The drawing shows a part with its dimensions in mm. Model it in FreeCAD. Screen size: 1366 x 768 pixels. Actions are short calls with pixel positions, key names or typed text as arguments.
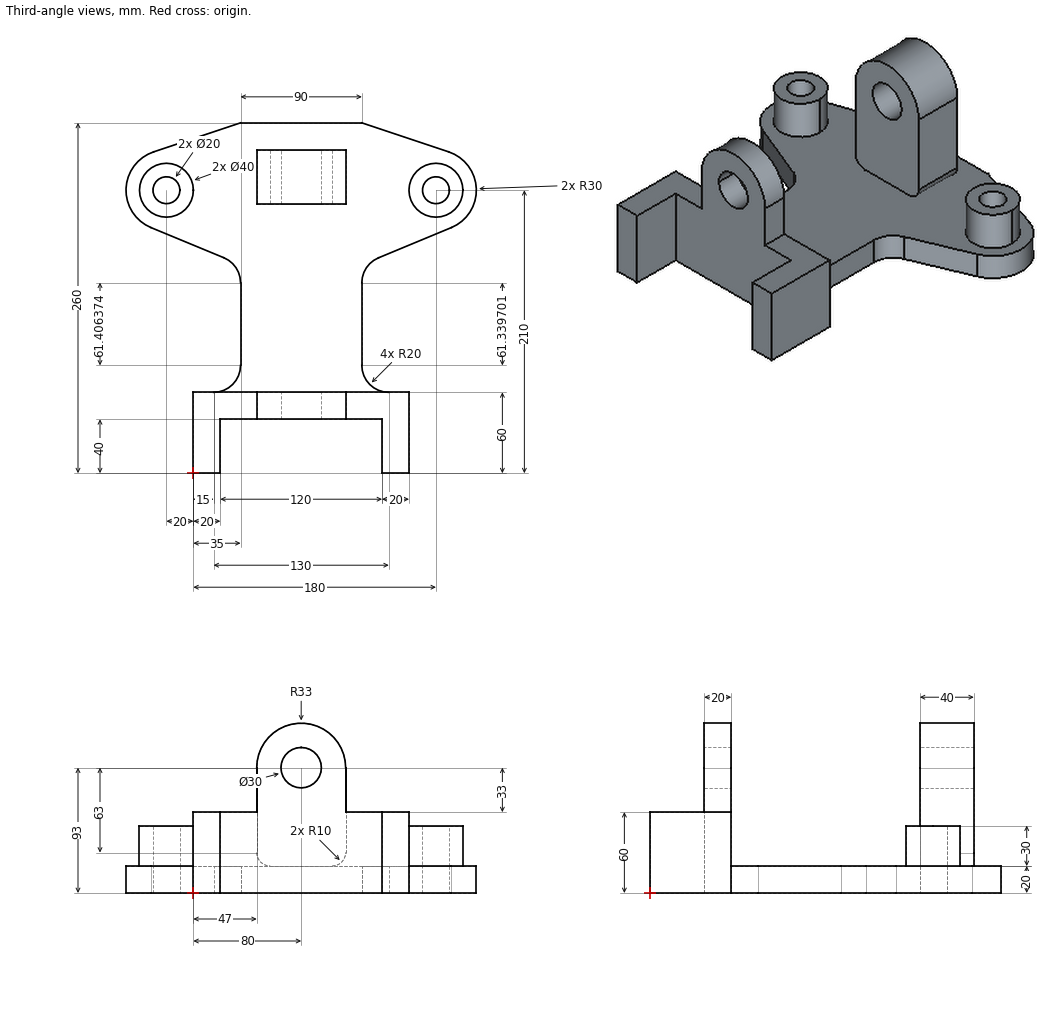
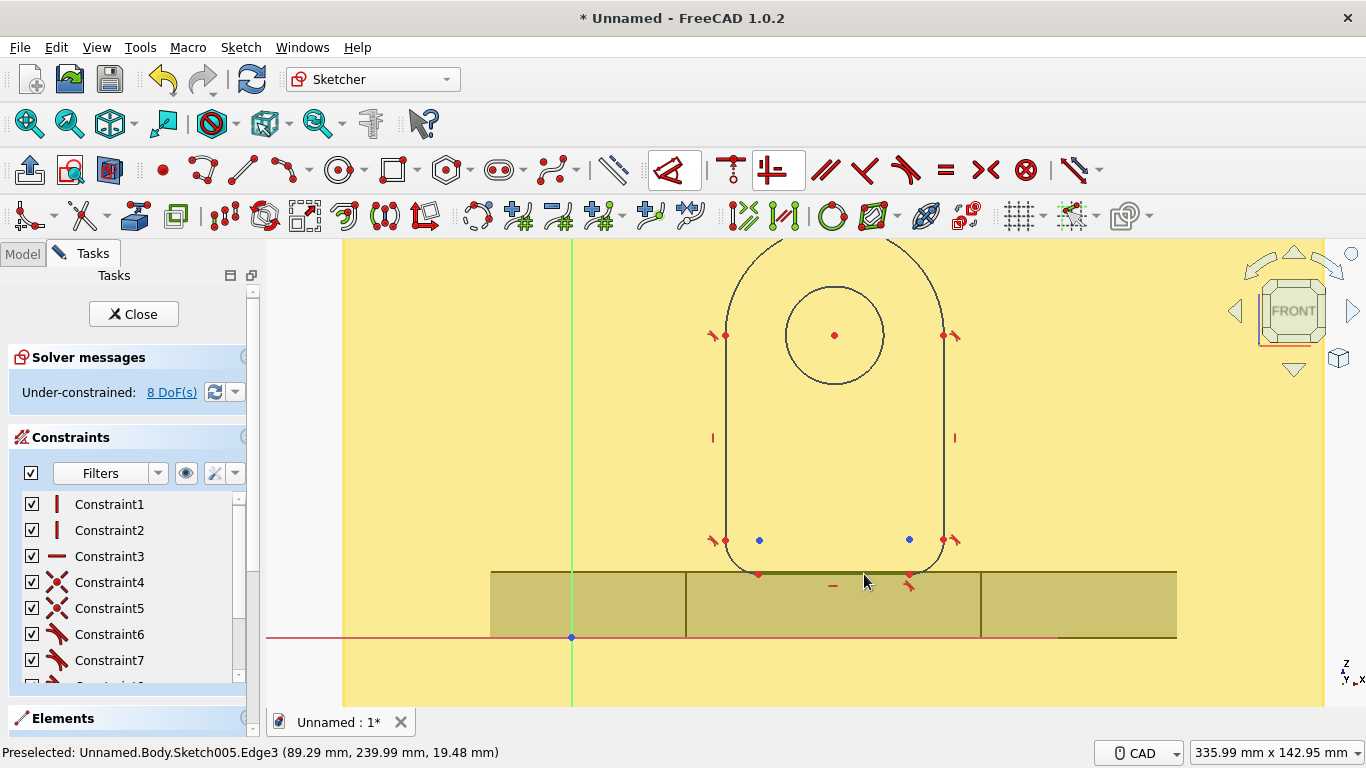
click(729, 555)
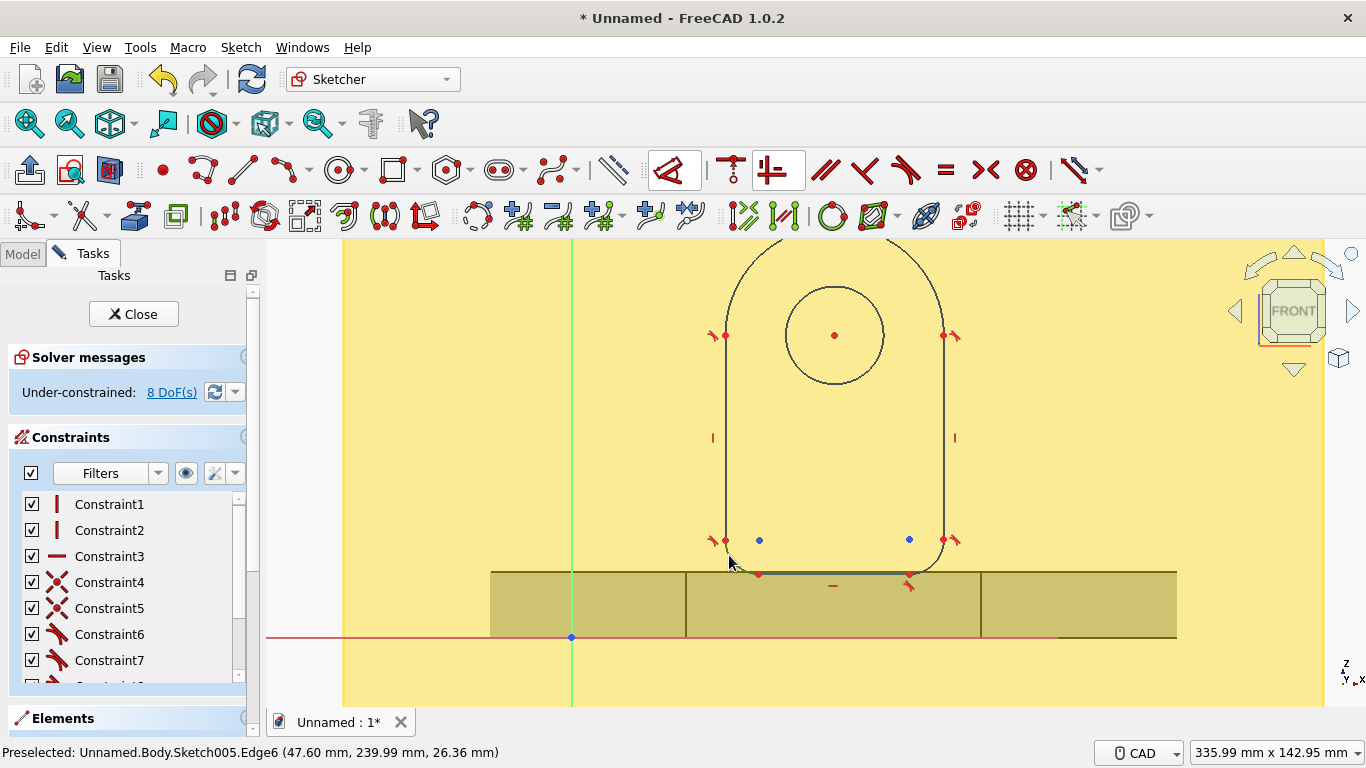
key(t)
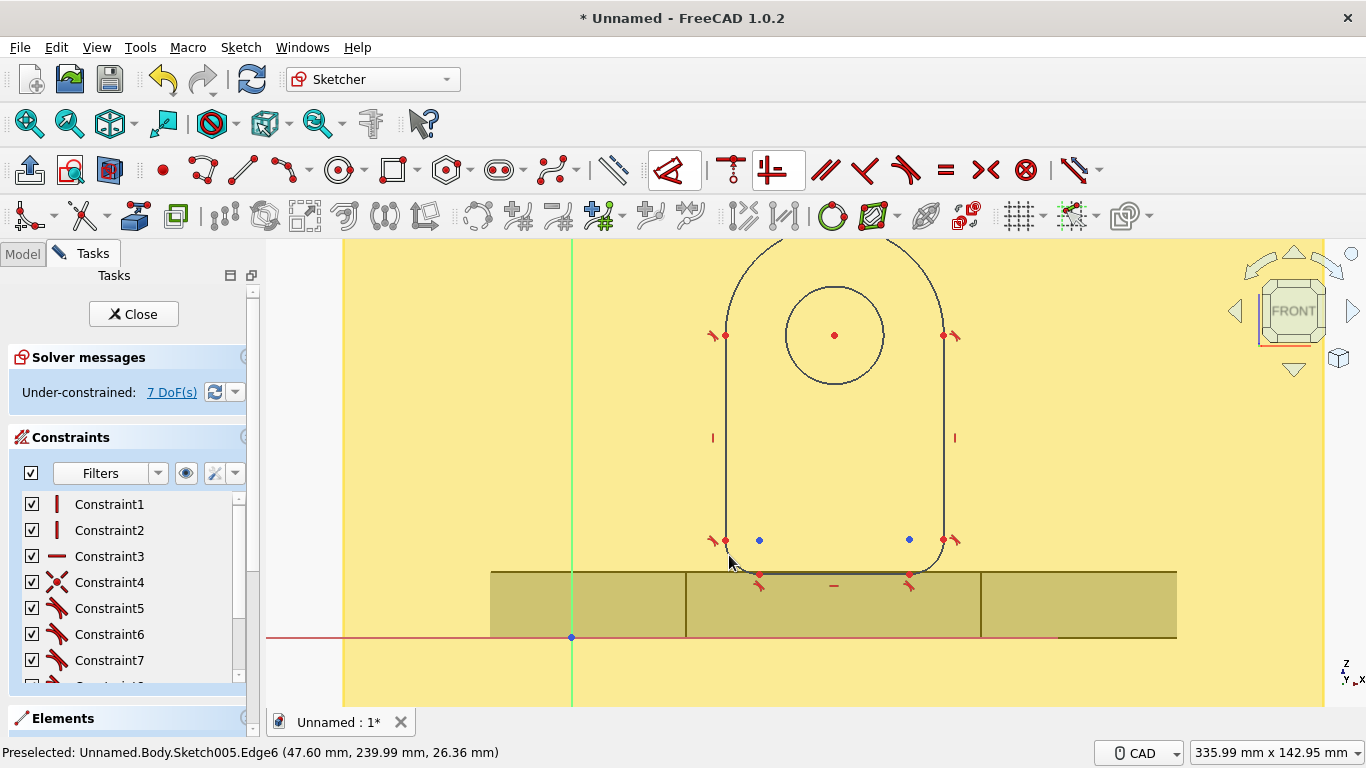
click(925, 570)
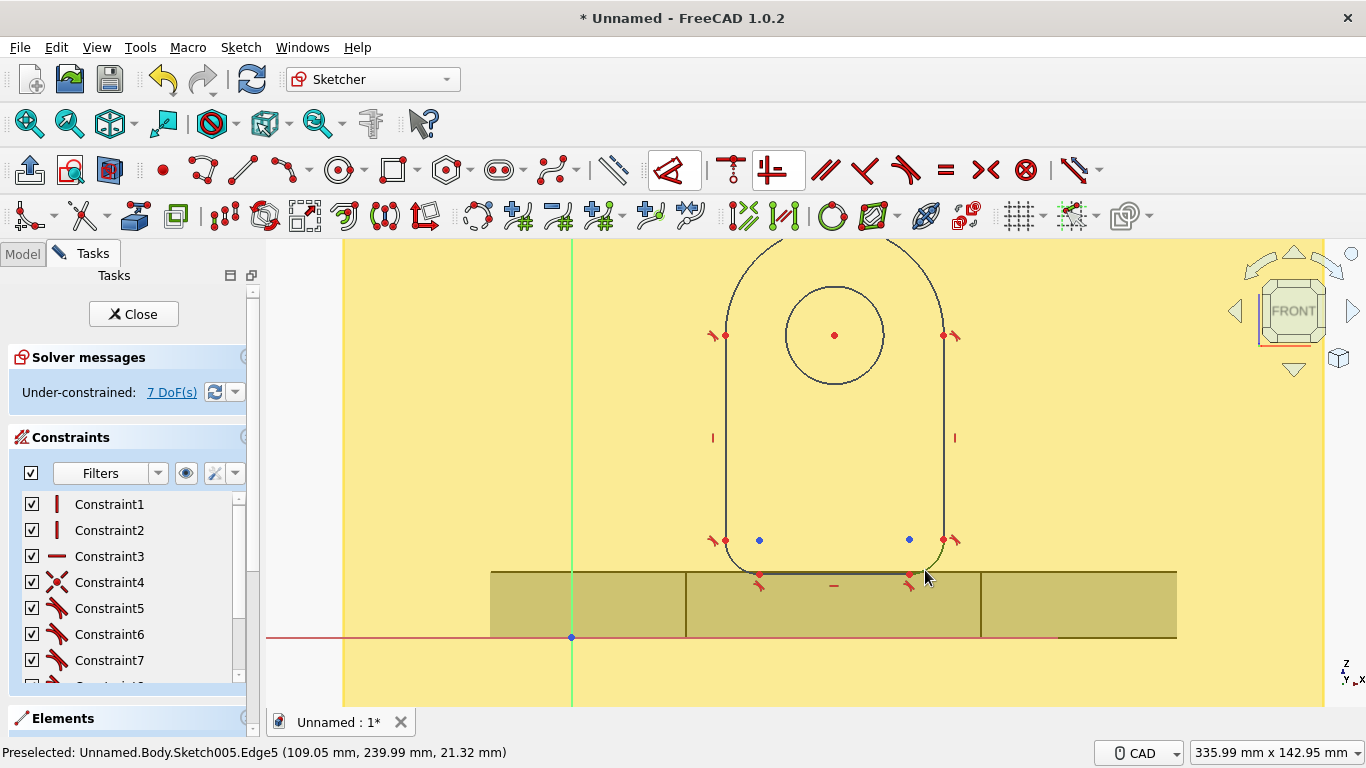
click(729, 556)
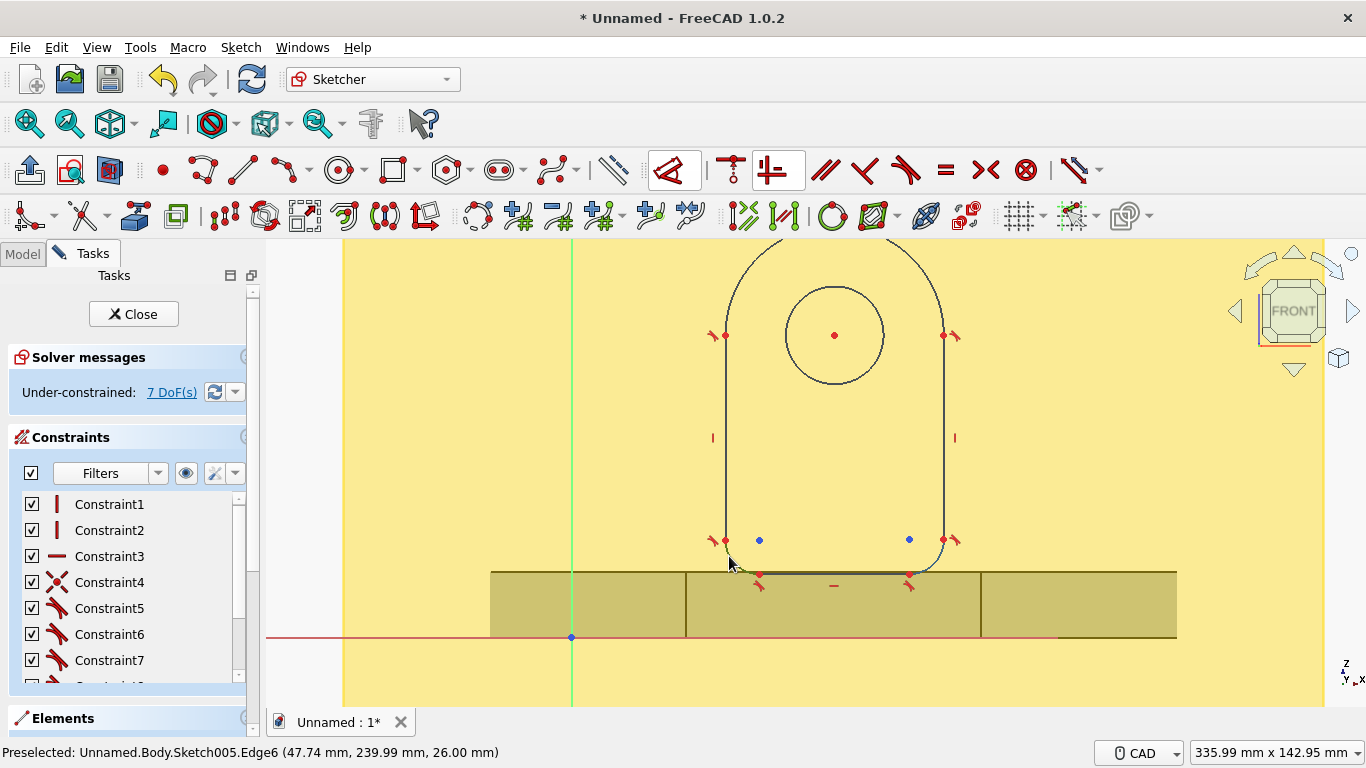
click(946, 170)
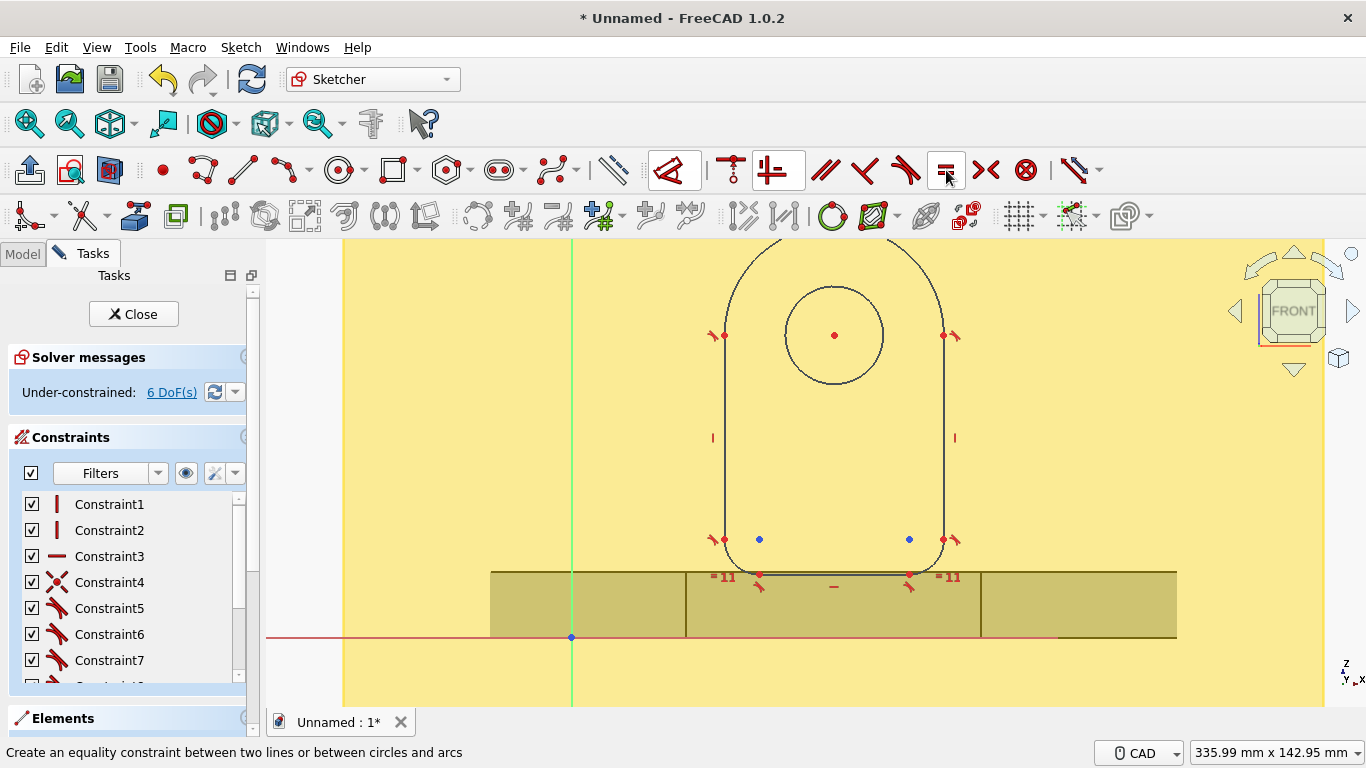
click(923, 271)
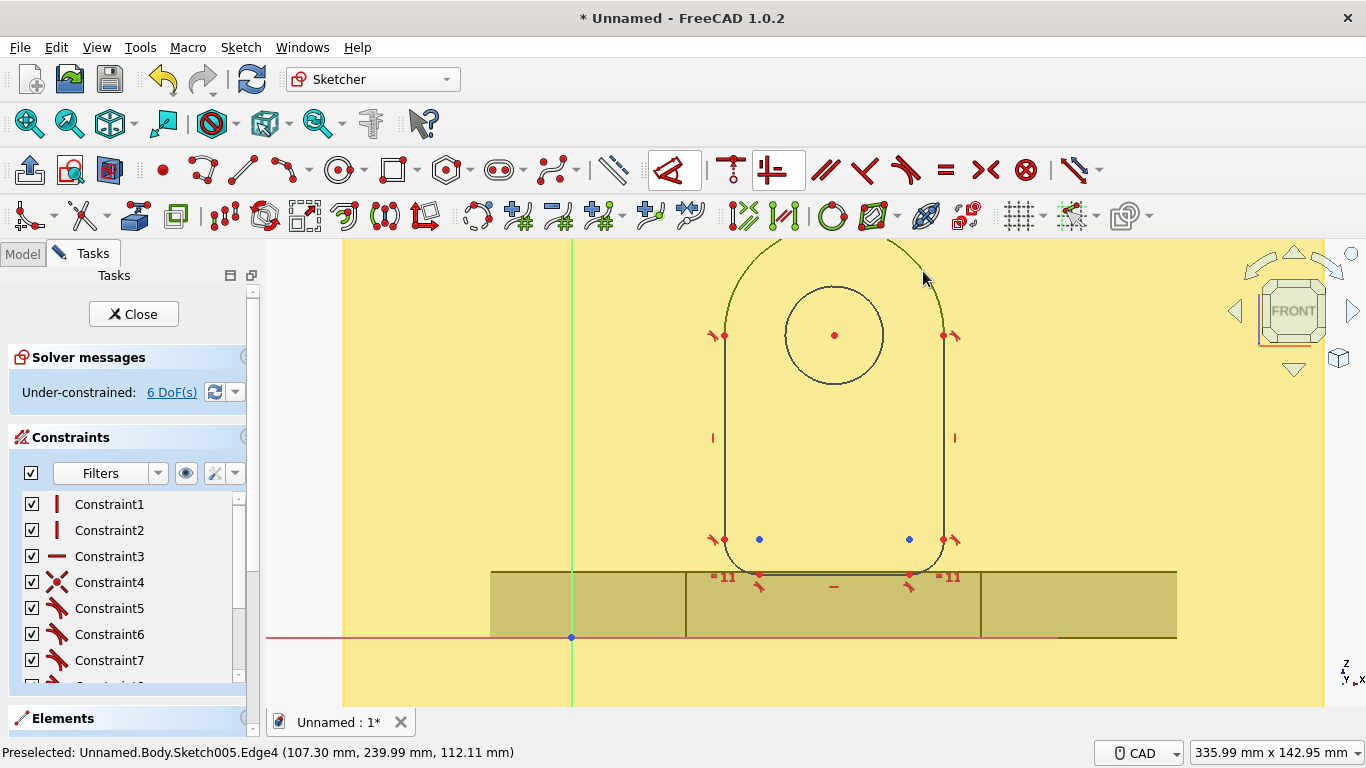
click(696, 170)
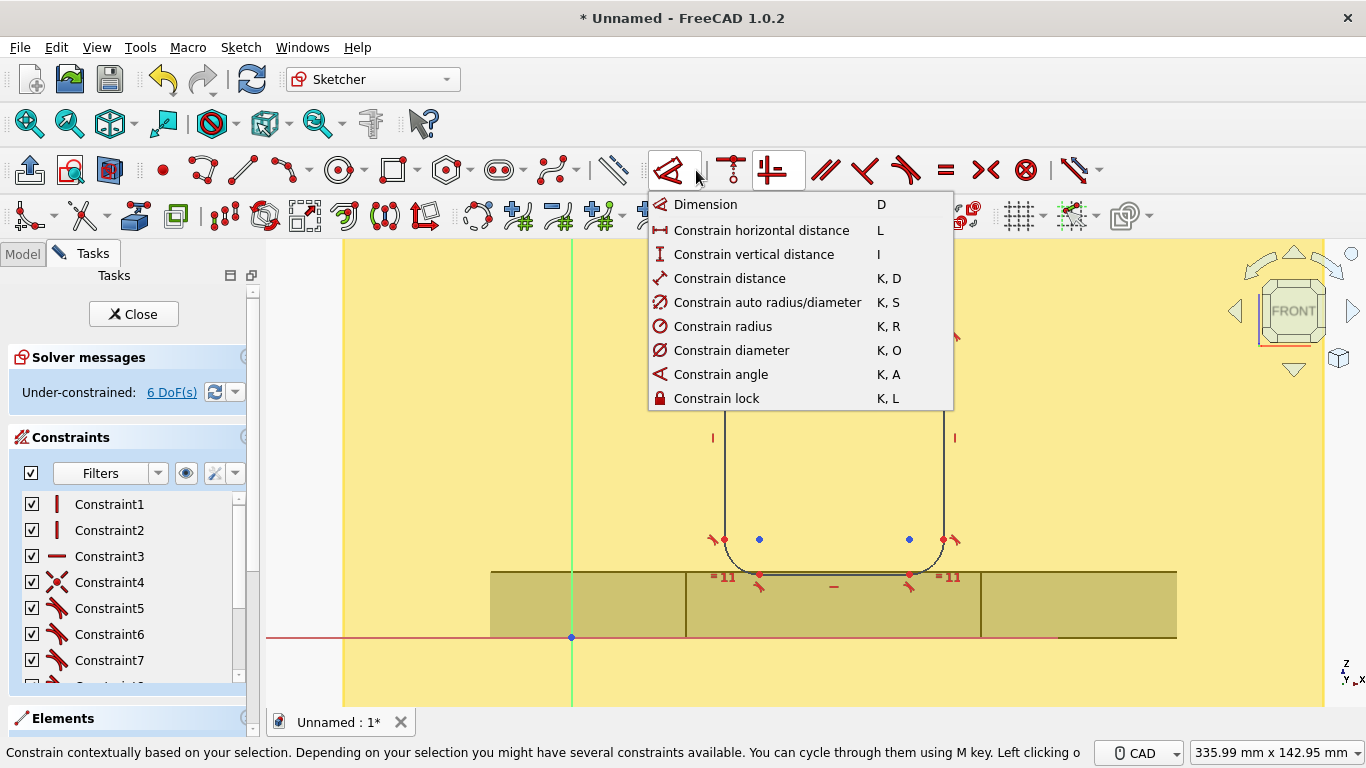
click(801, 326)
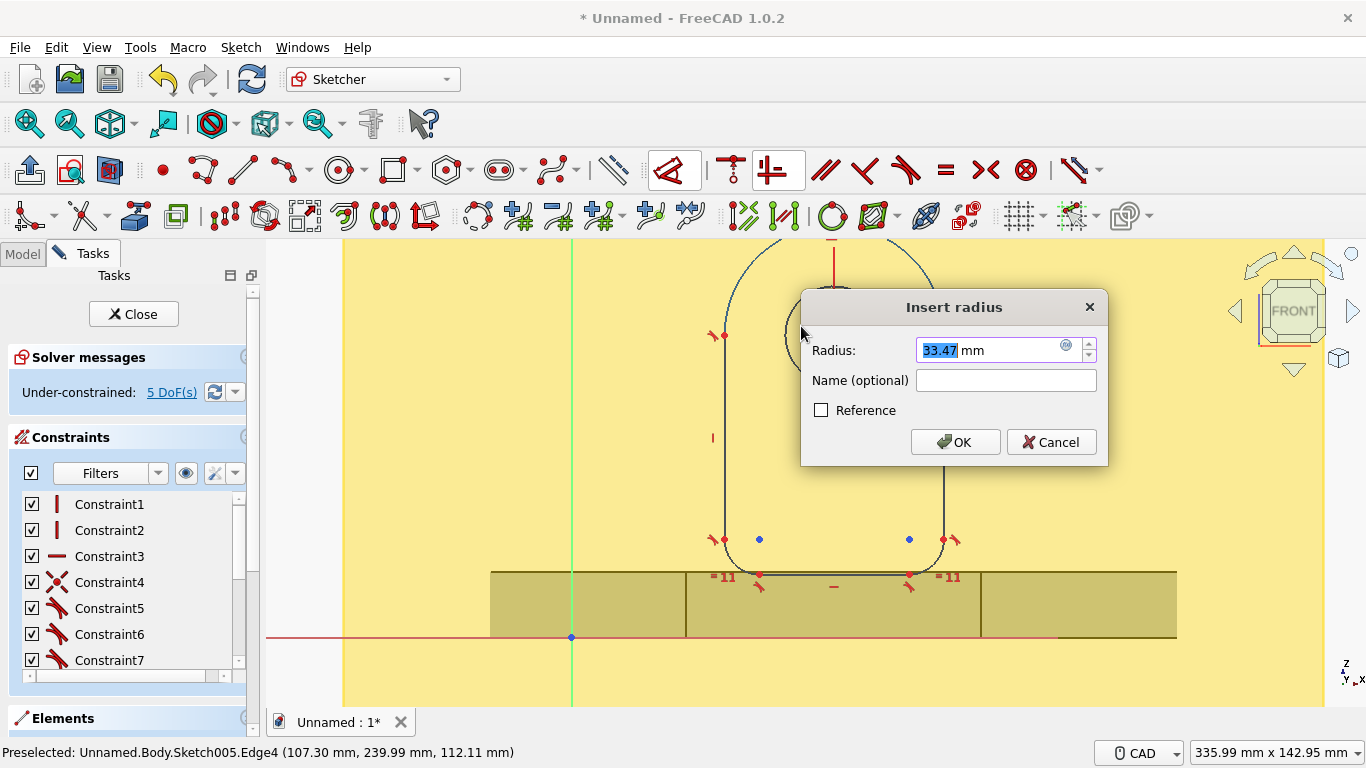
text(33)
key(Return)